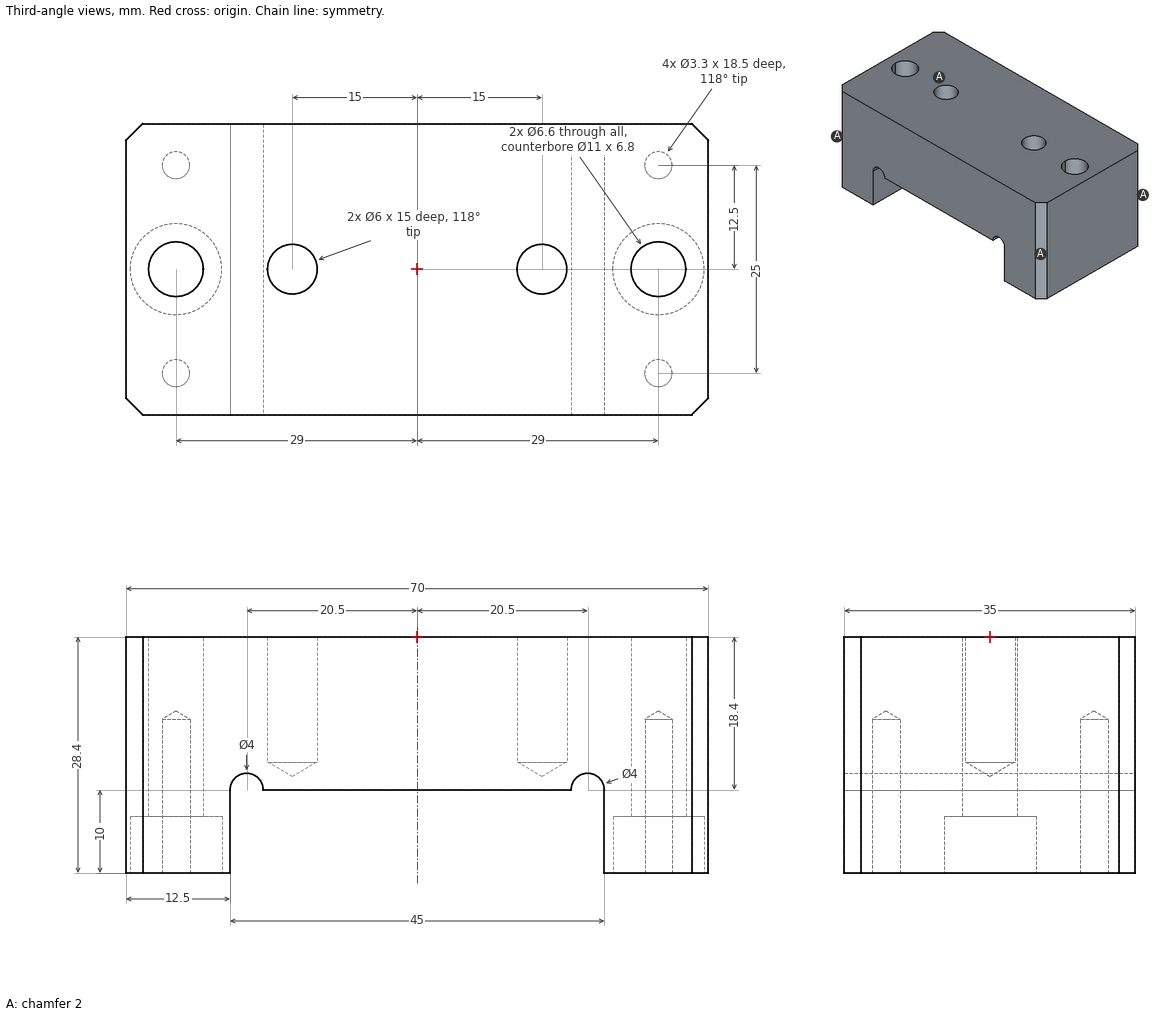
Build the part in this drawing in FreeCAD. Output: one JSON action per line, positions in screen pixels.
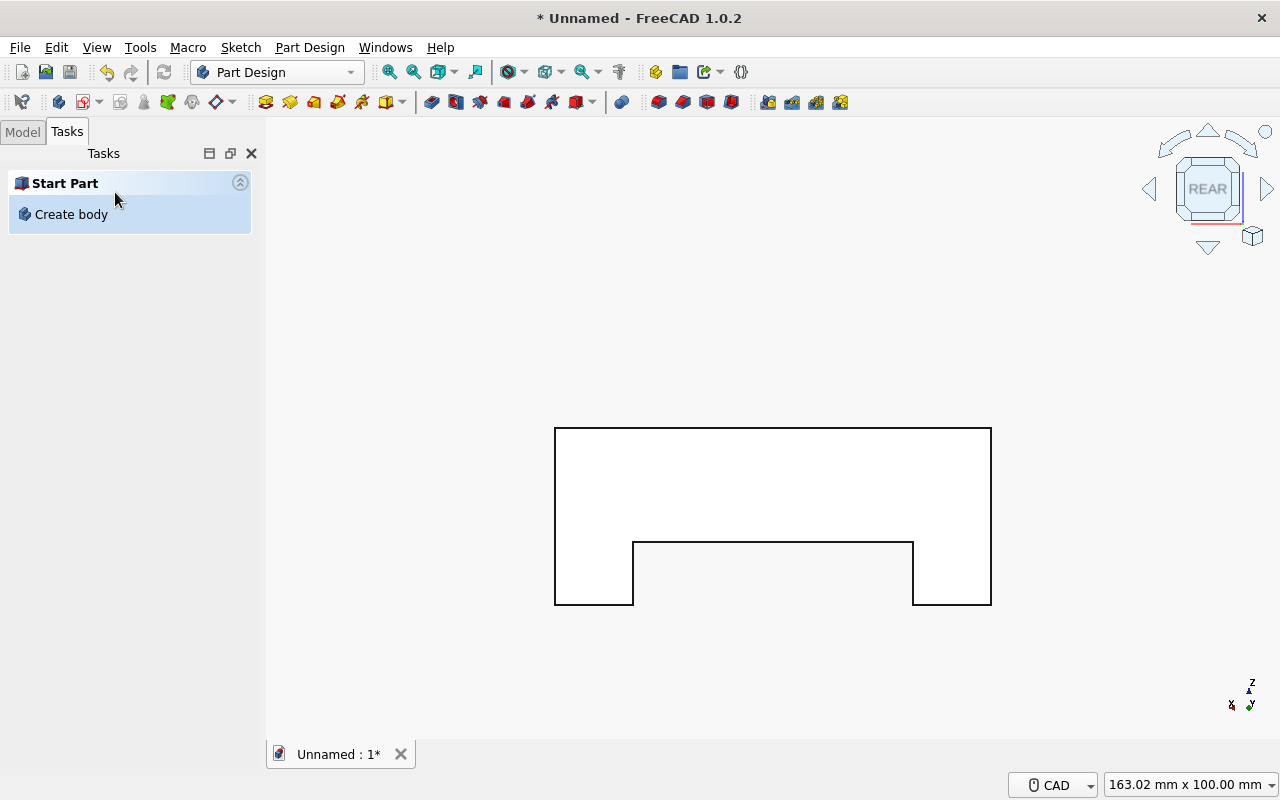
{"action": "key", "text": "v f"}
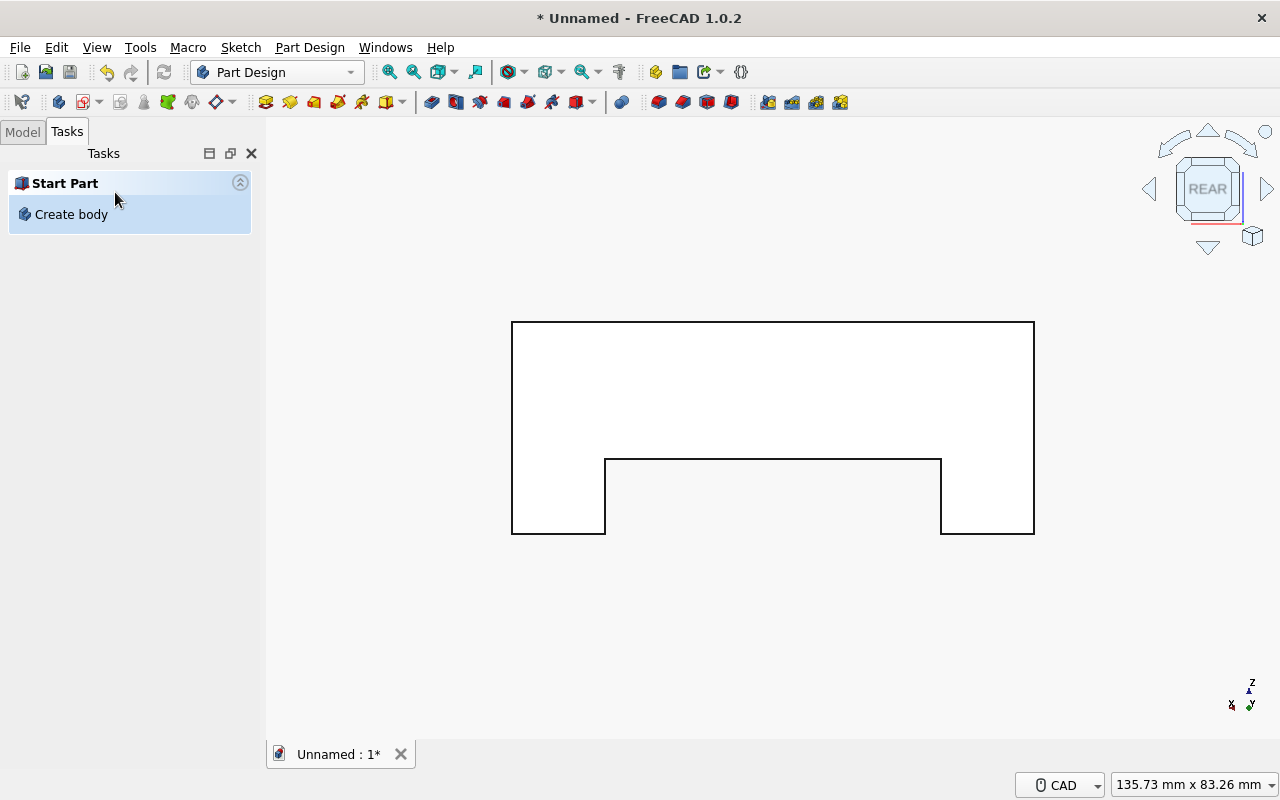
{"action": "left_click", "coordinate": [624, 397]}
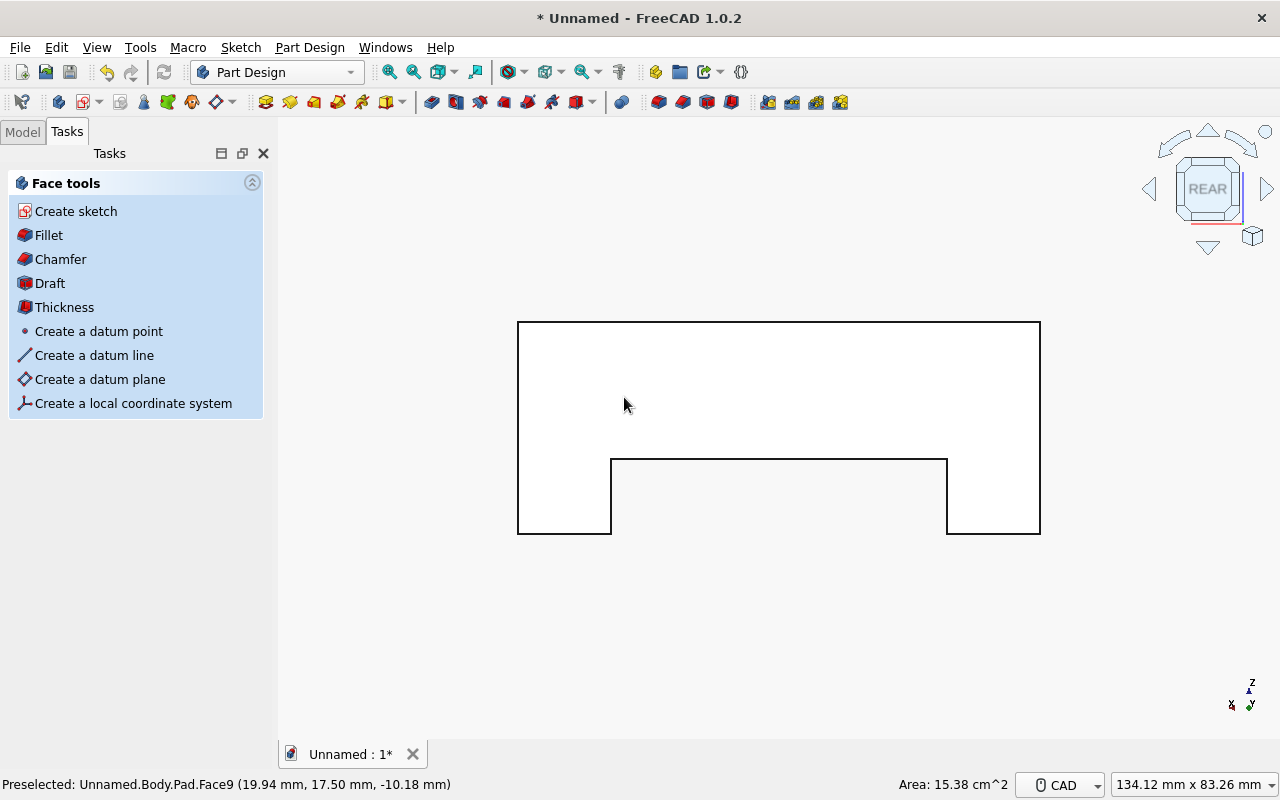
{"action": "left_click", "coordinate": [84, 102]}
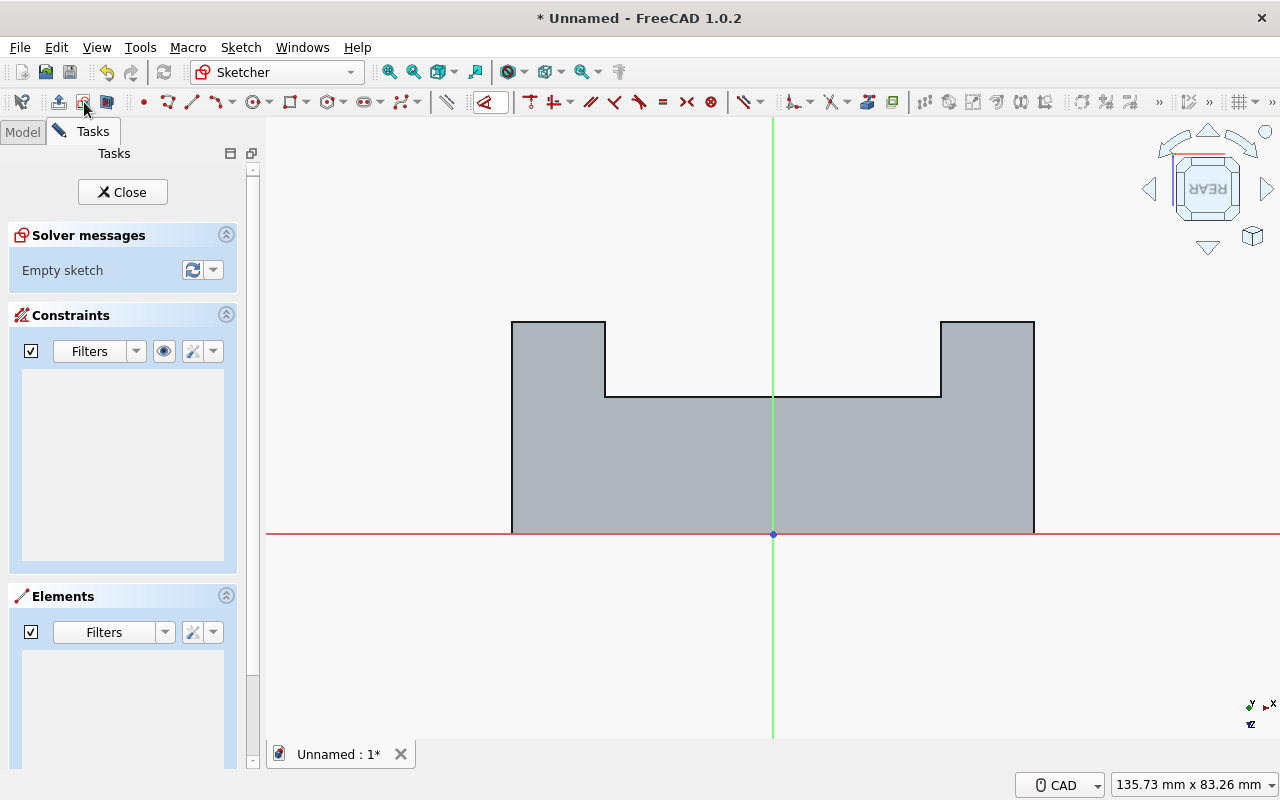
{"action": "scroll", "coordinate": [944, 394], "scroll_direction": "up", "scroll_amount": 13}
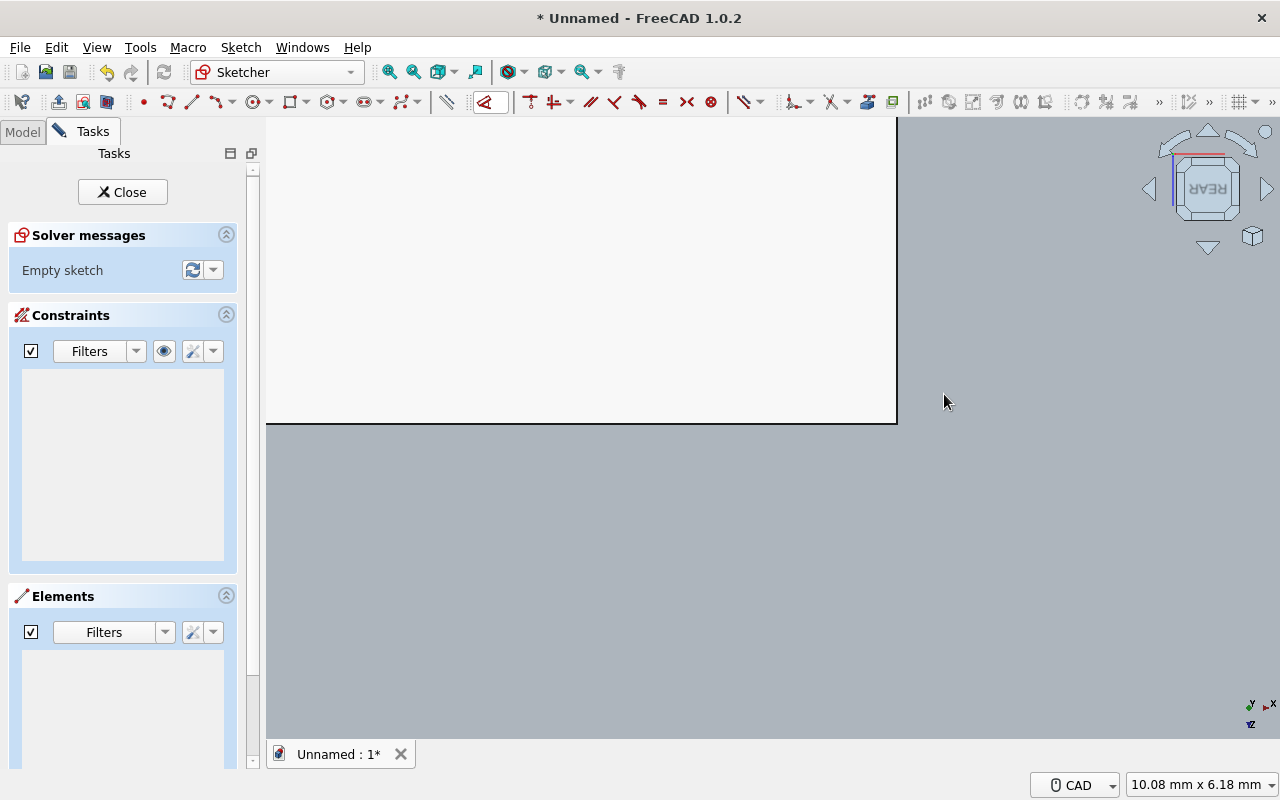
{"action": "key", "text": "g c"}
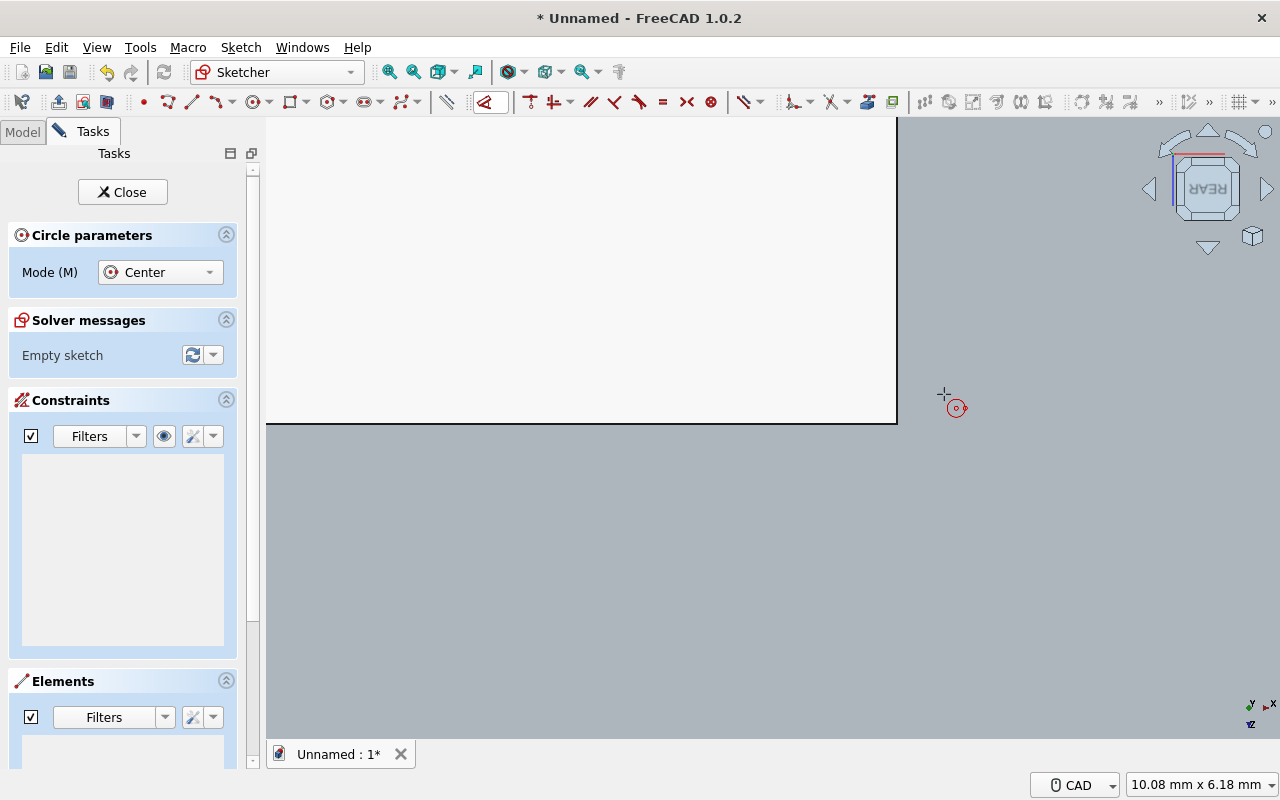
{"action": "left_click", "coordinate": [695, 424]}
{"action": "left_click", "coordinate": [838, 281]}
{"action": "key", "text": "Escape"}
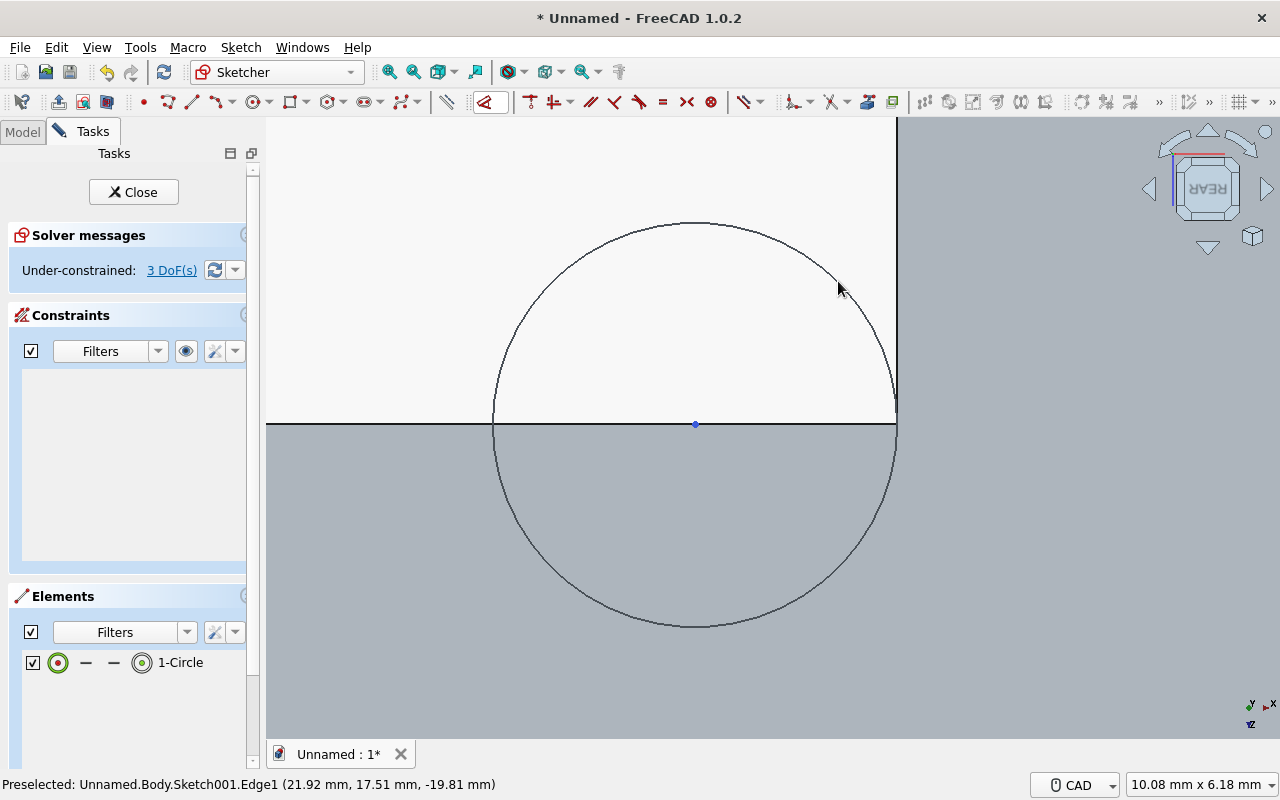
{"action": "key", "text": "d"}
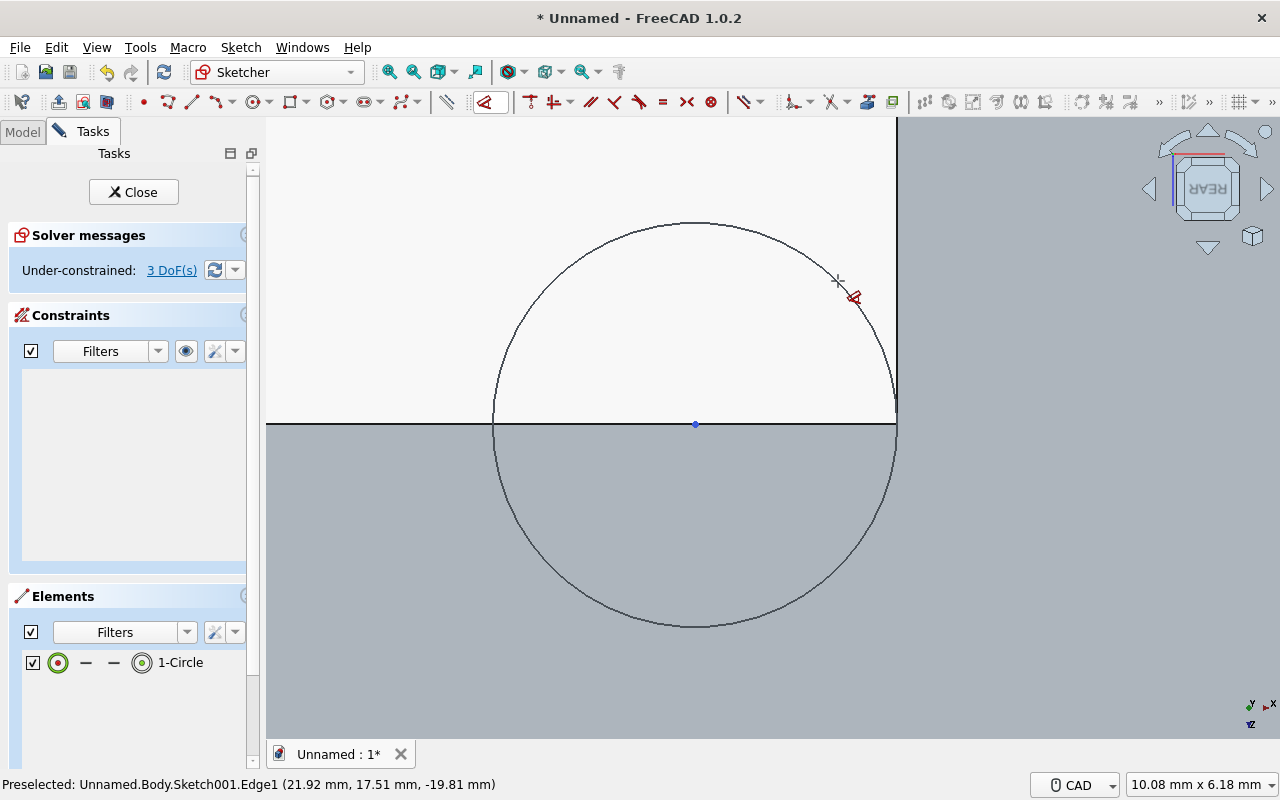
{"action": "left_click", "coordinate": [838, 282]}
{"action": "left_click", "coordinate": [861, 259]}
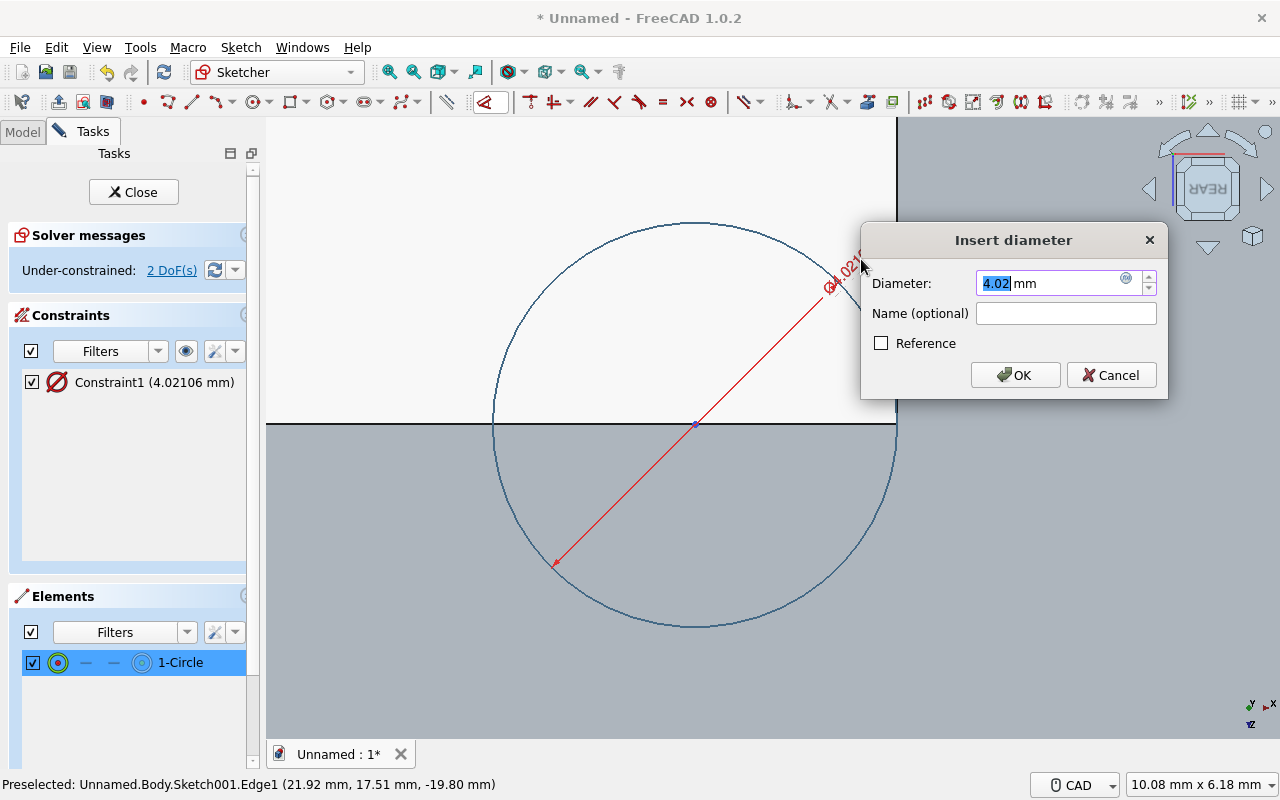
{"action": "type", "text": "4"}
{"action": "key", "text": "Return"}